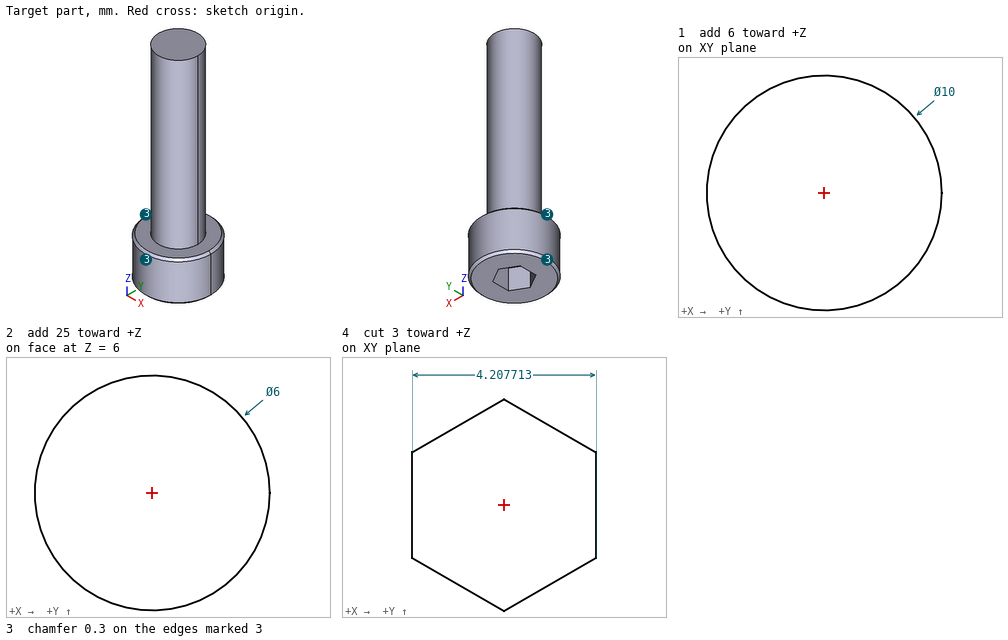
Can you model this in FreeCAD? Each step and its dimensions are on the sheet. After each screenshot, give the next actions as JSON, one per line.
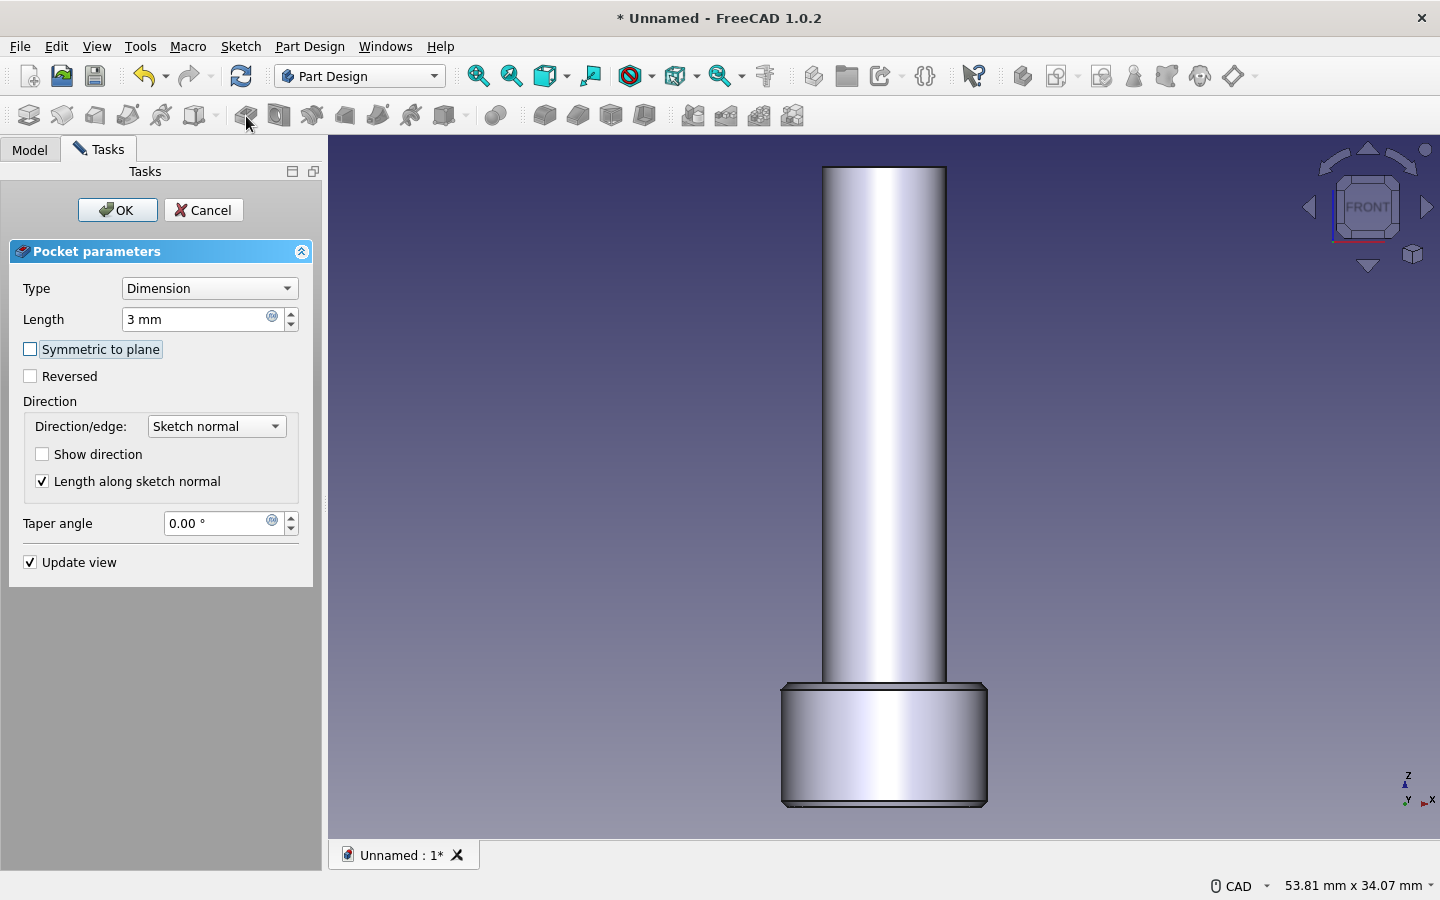
{"action": "left_click", "coordinate": [31, 376]}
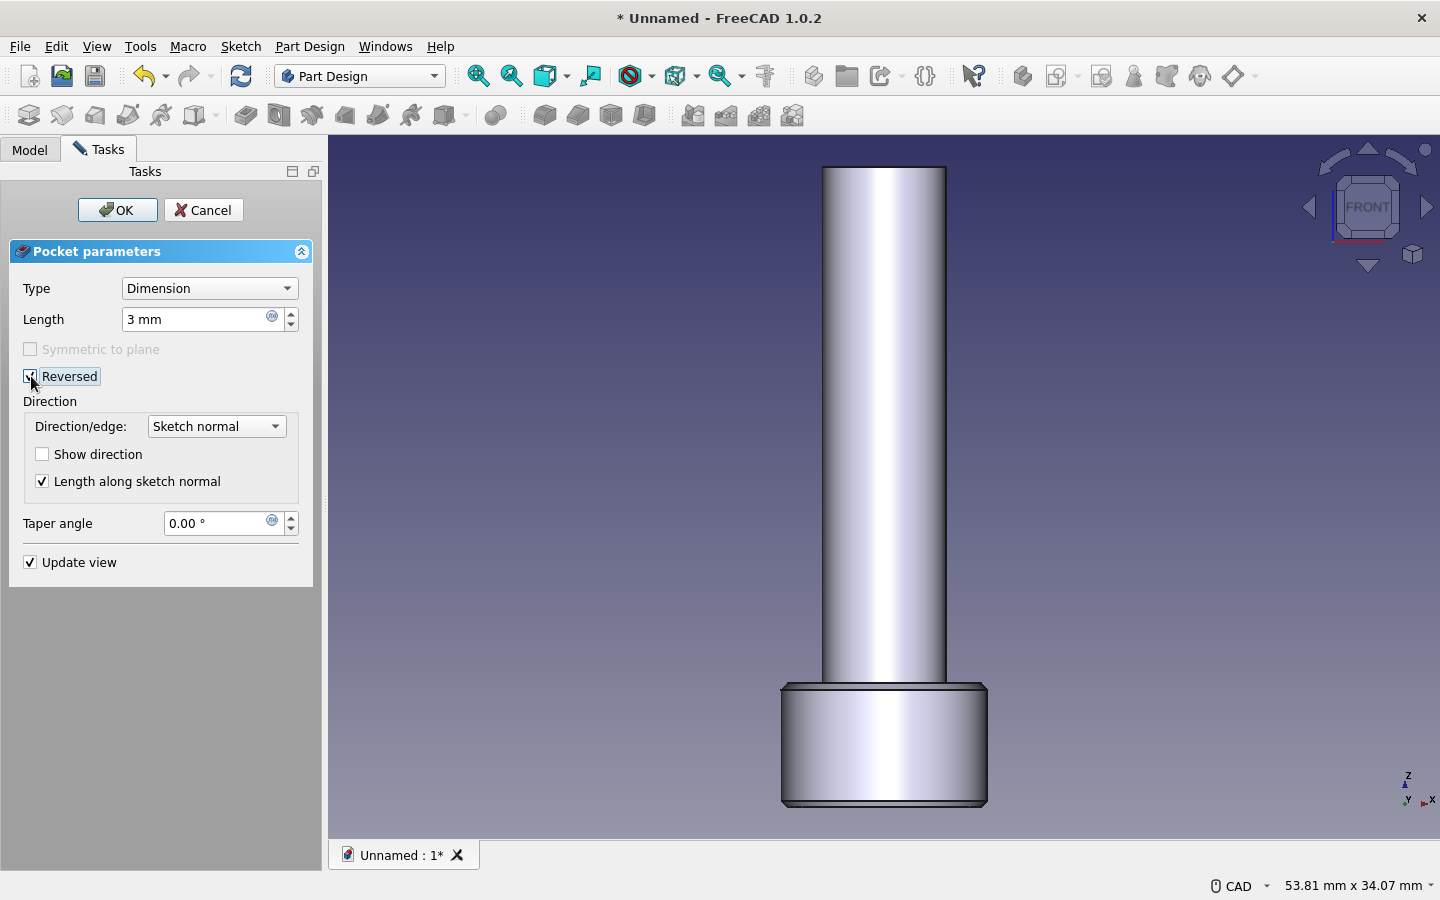
{"action": "left_click", "coordinate": [118, 210]}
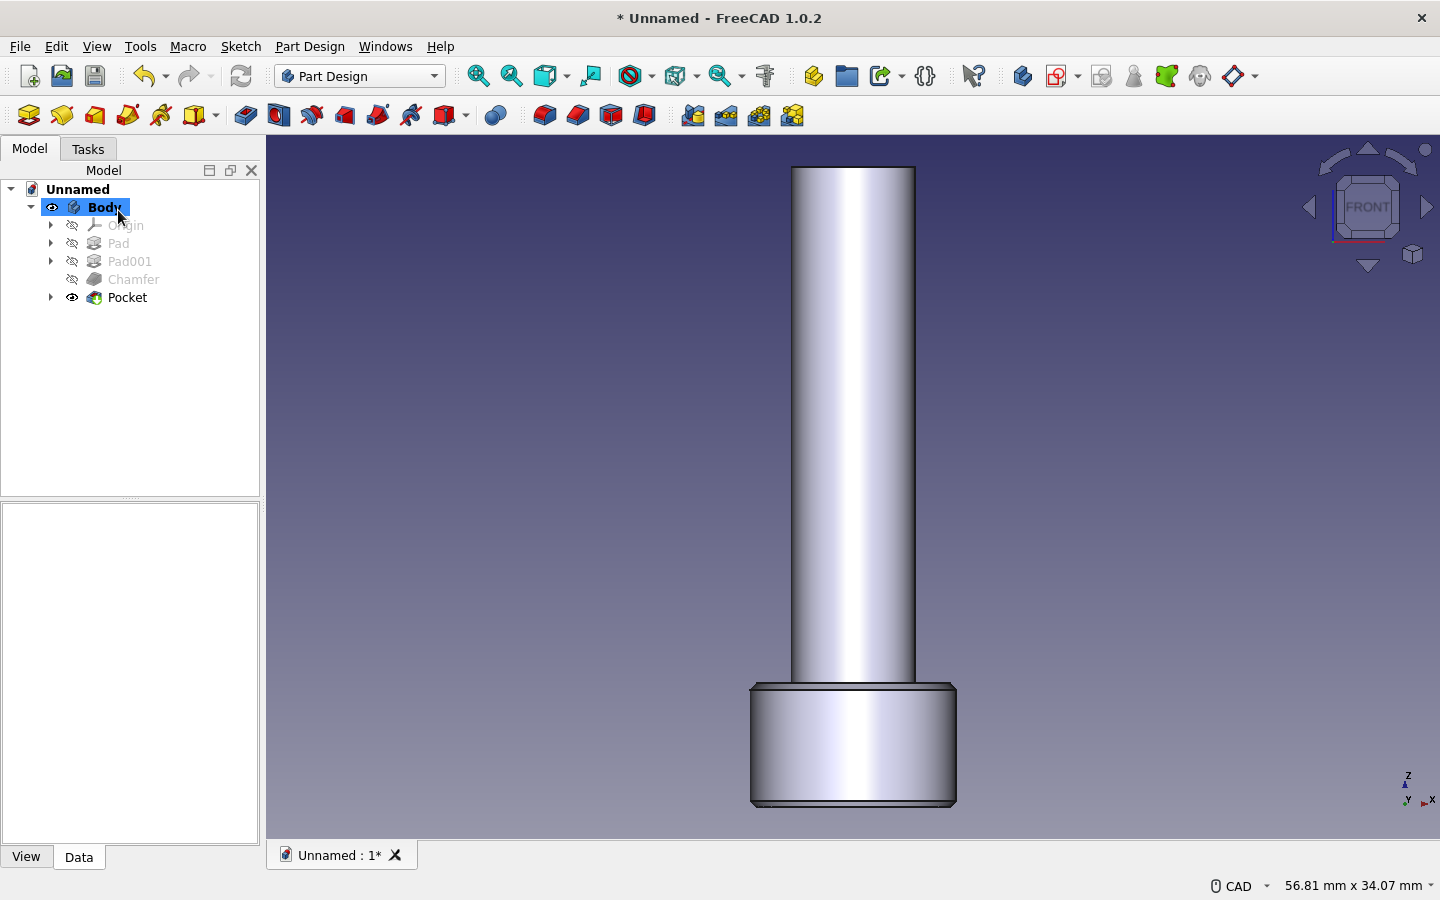
{"action": "key", "text": "0"}